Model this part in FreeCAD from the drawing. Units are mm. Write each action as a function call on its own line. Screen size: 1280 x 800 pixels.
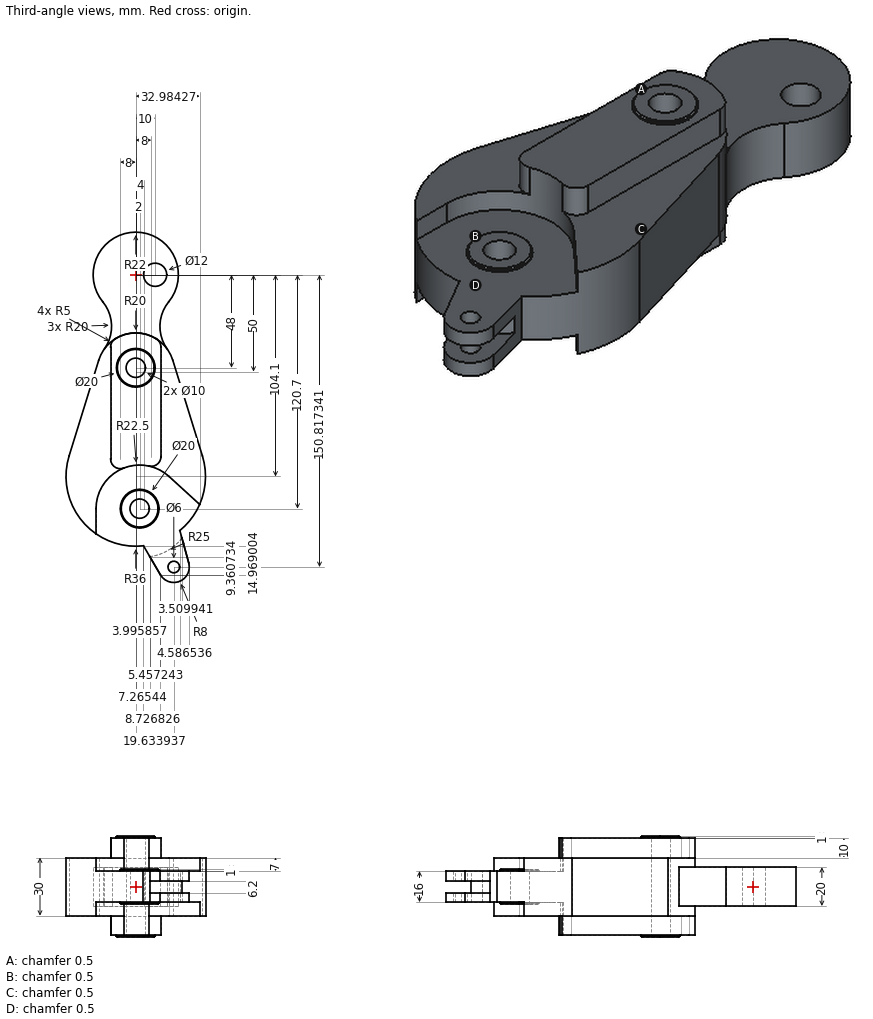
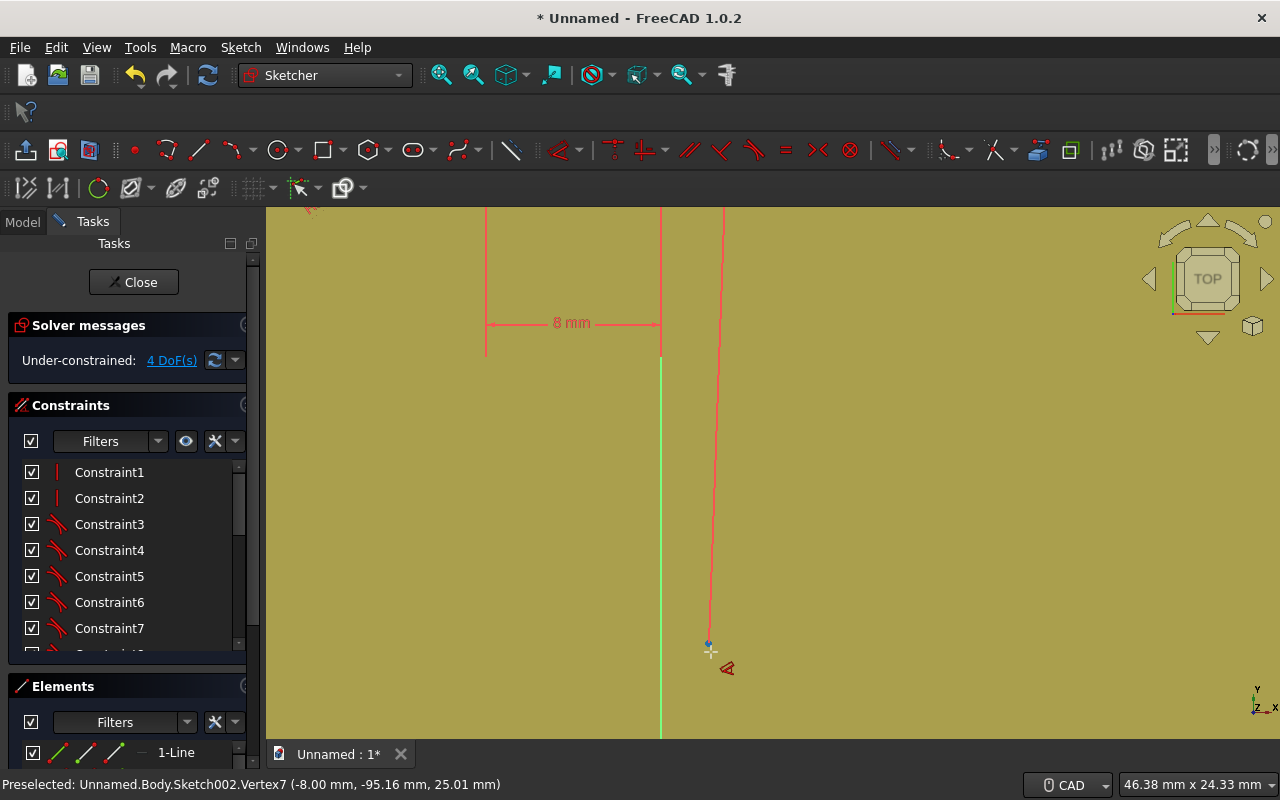
click(709, 643)
click(685, 677)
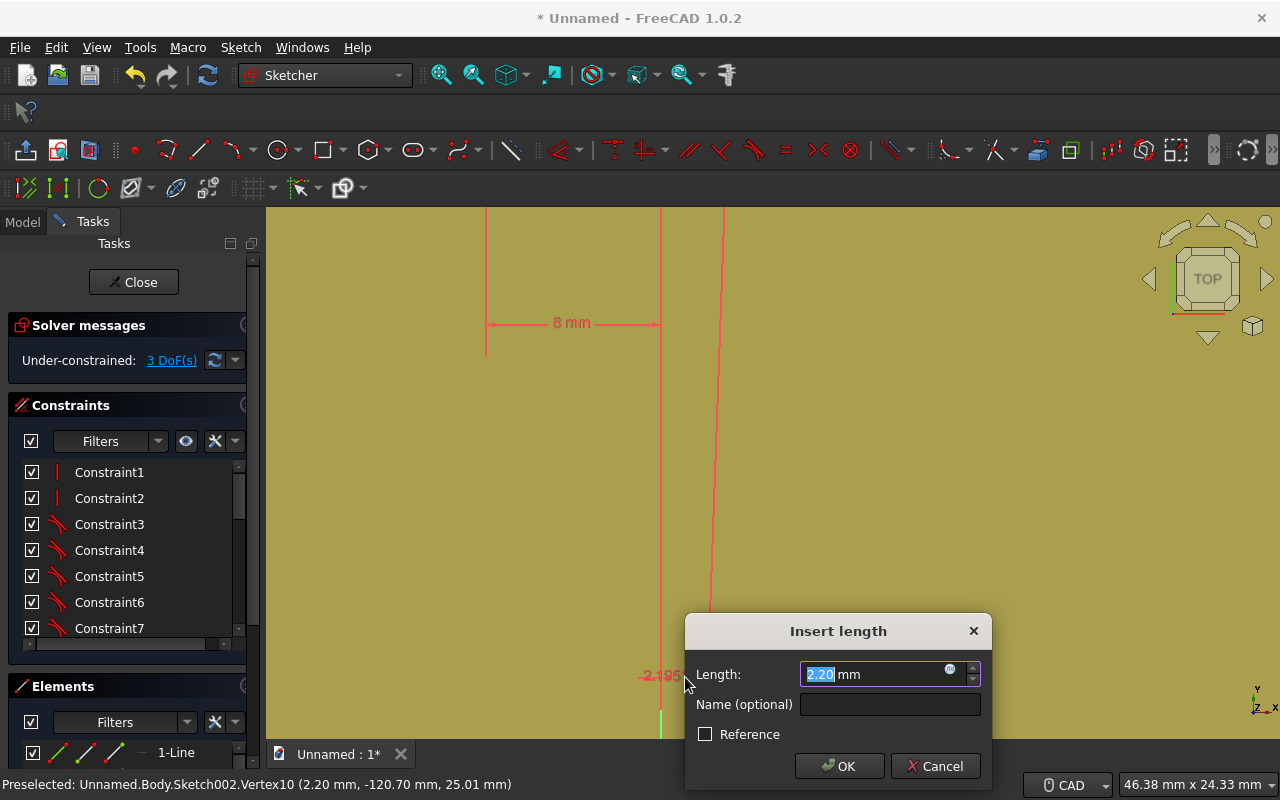
text(2)
key(Return)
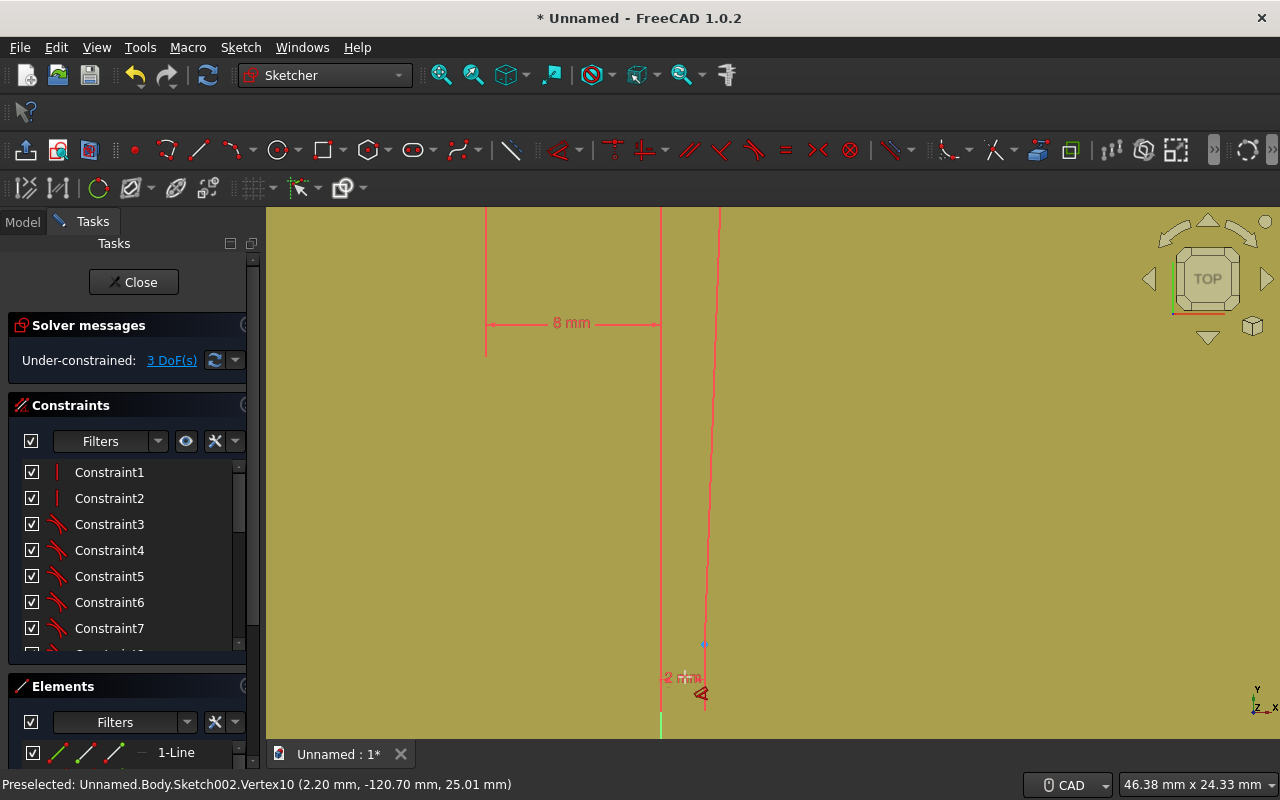
scroll(713, 711, down, 9)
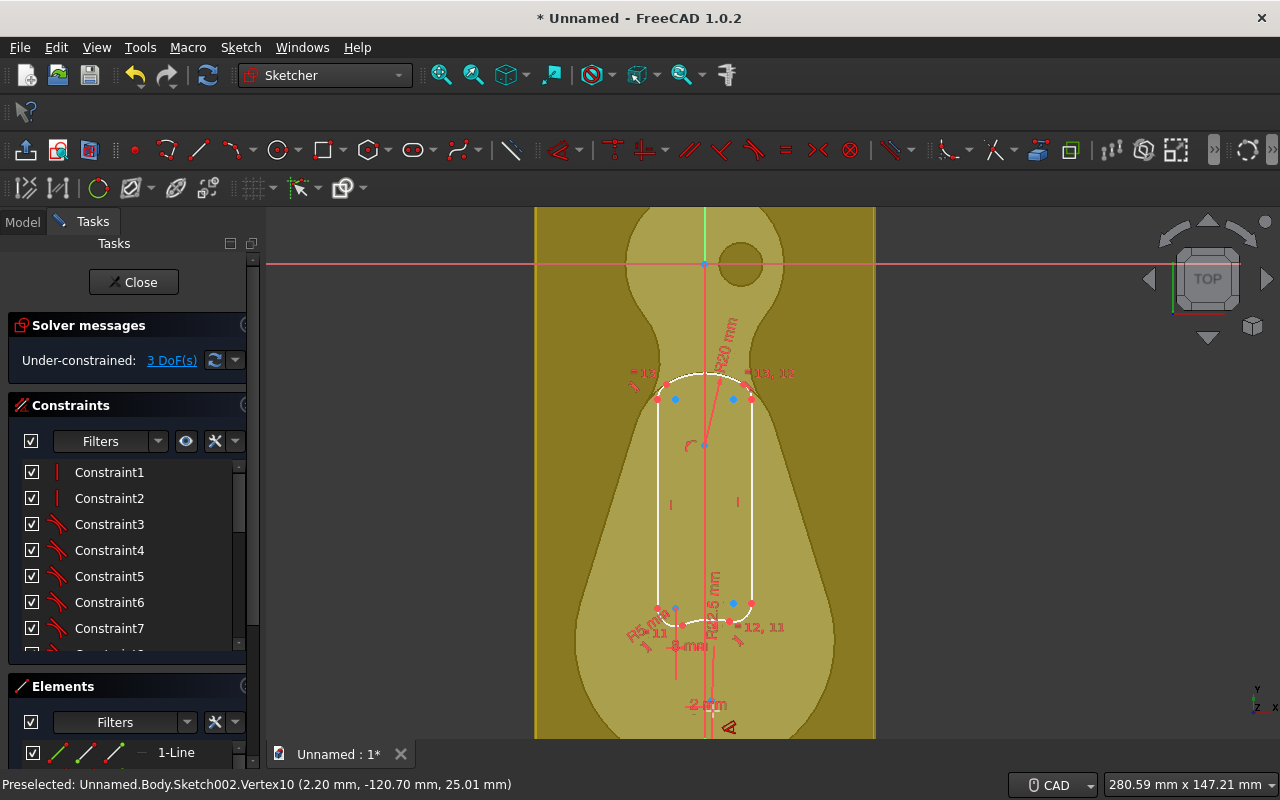
scroll(734, 604, up, 2)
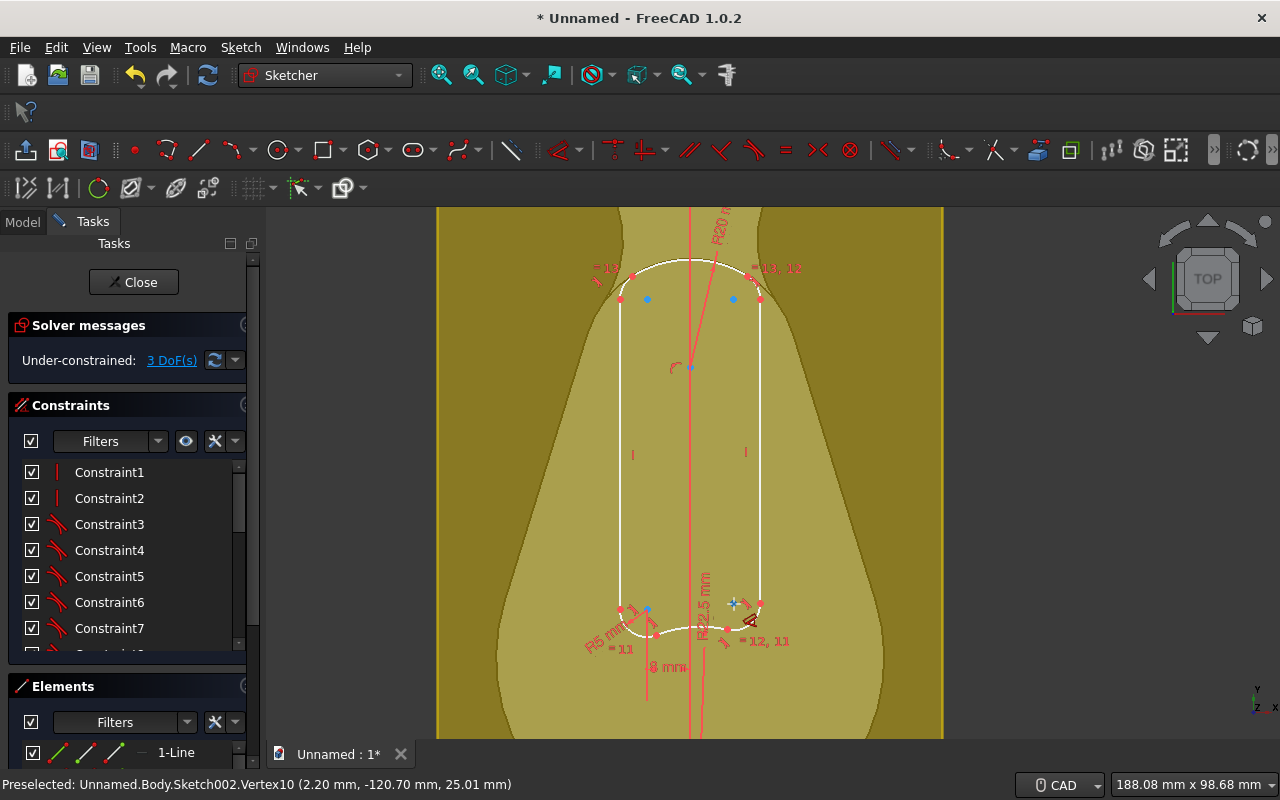
click(733, 603)
click(712, 709)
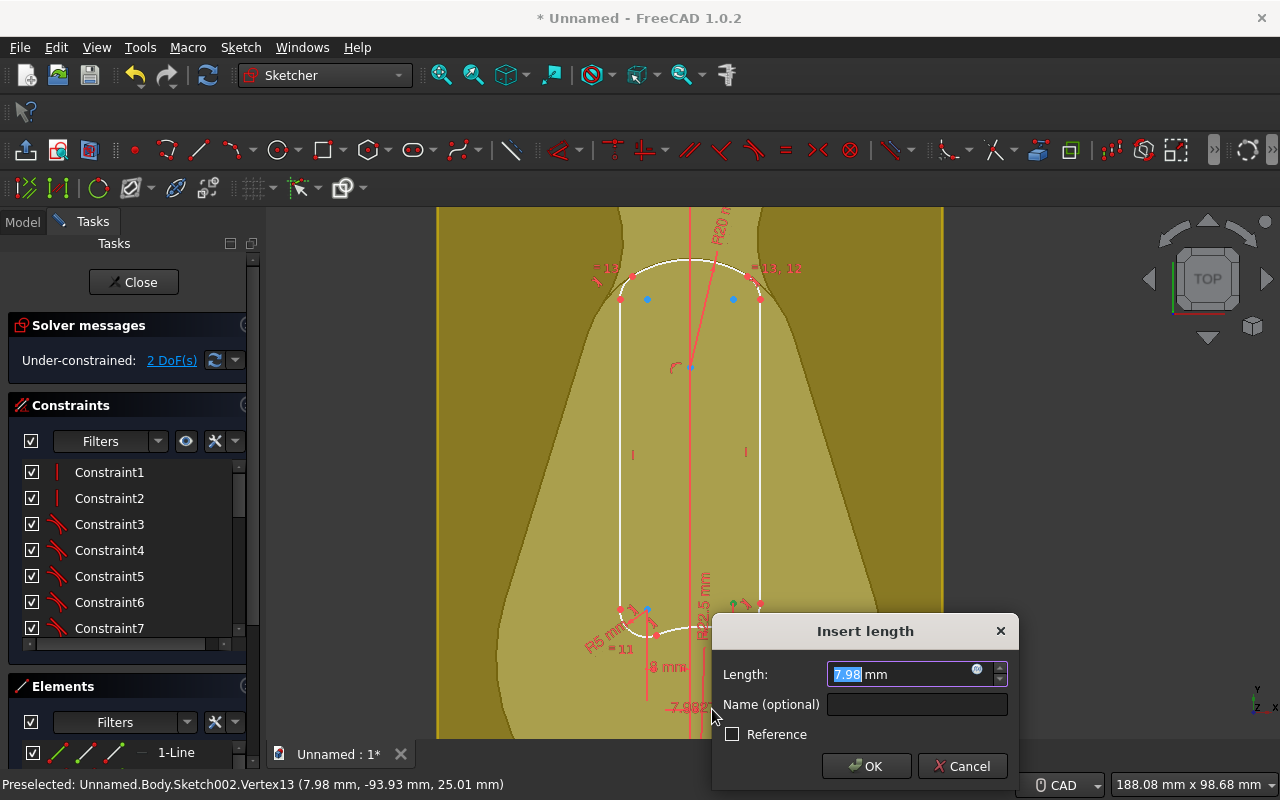
text(8)
key(Return)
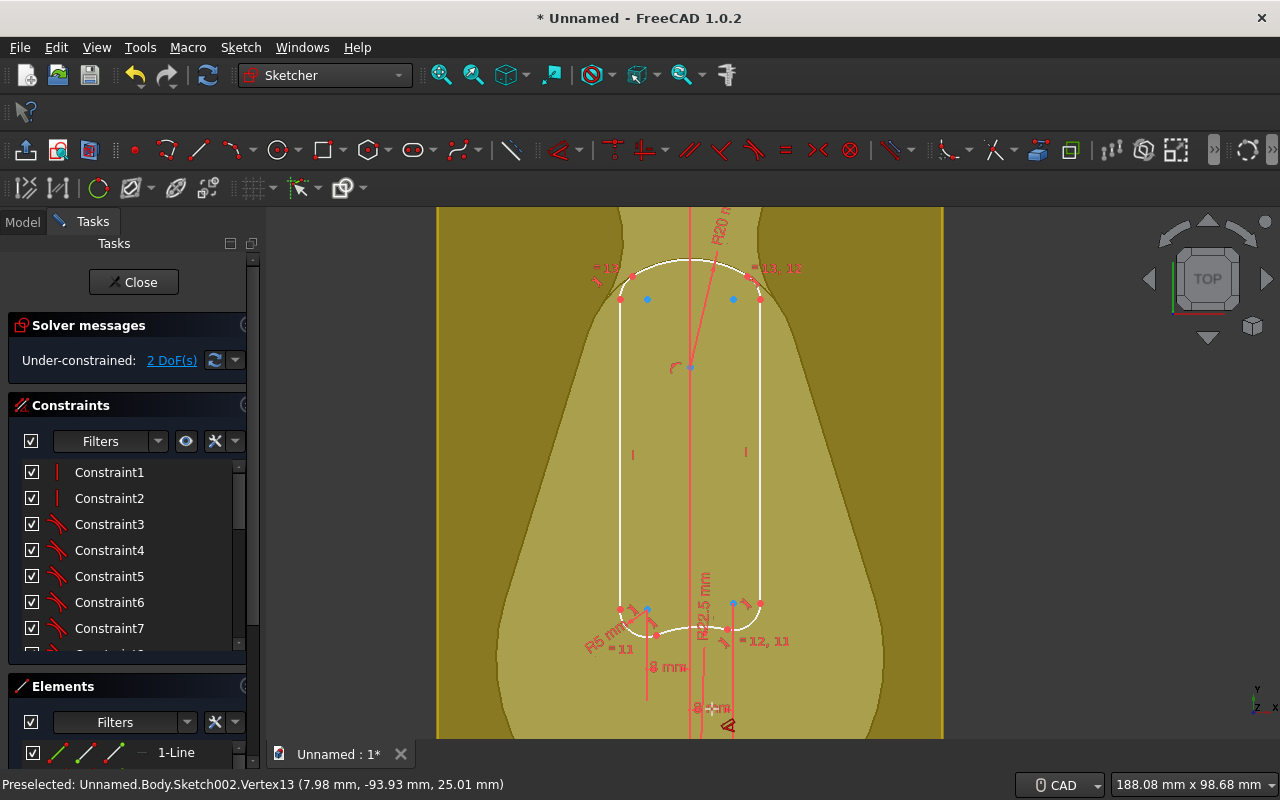
click(690, 368)
click(724, 301)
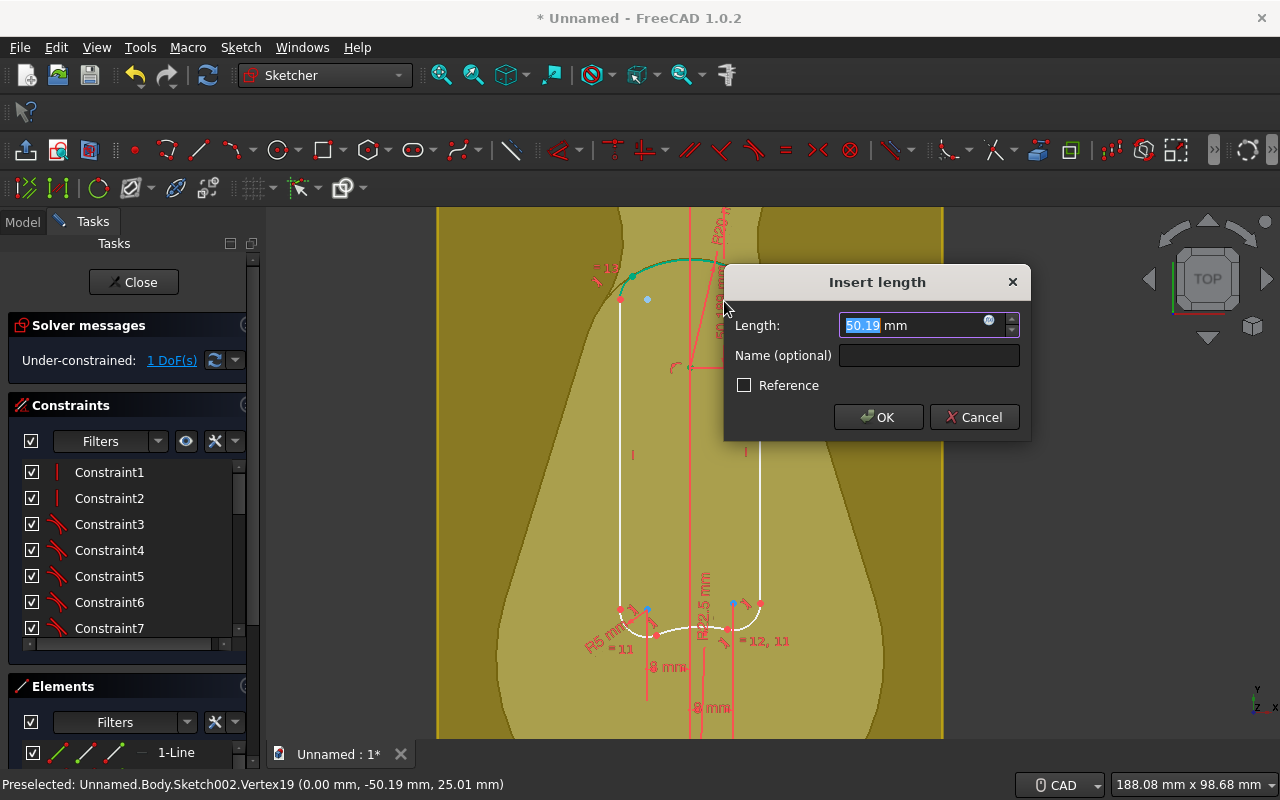
text(50)
key(Return)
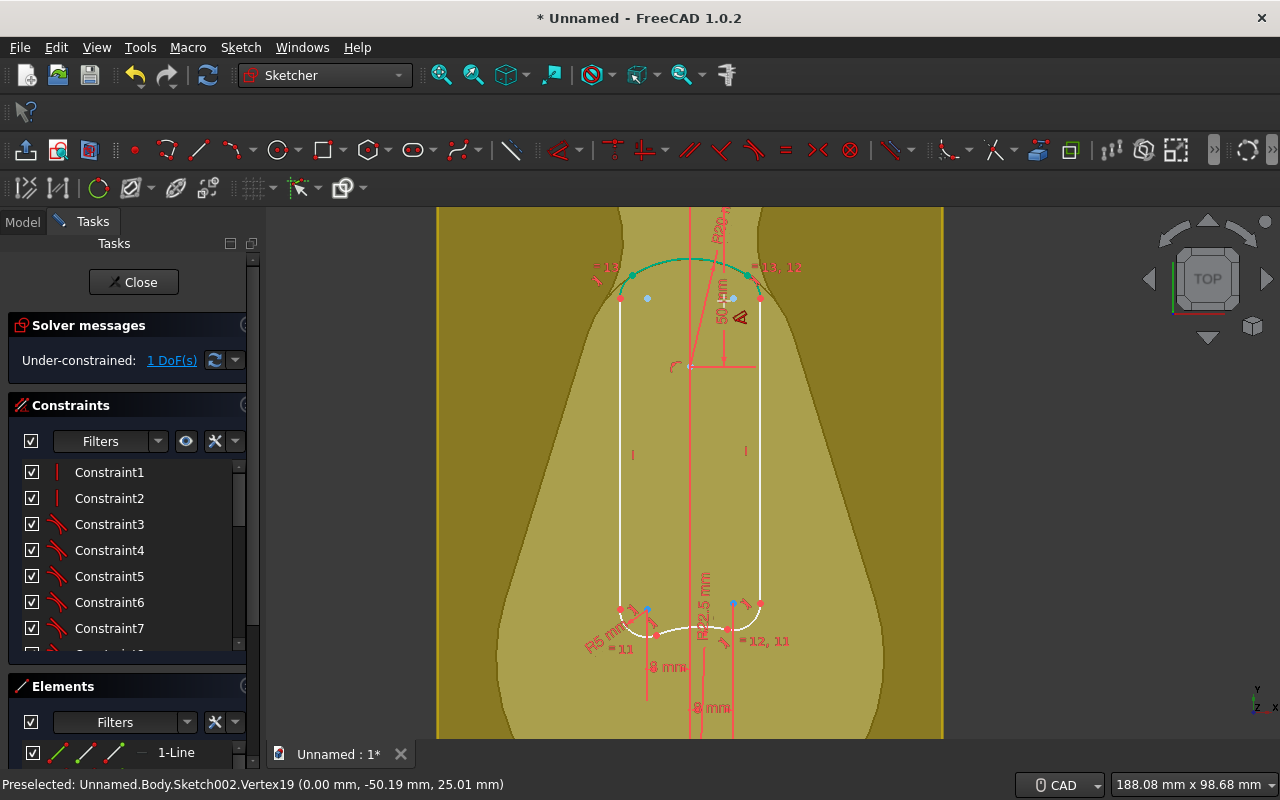
scroll(734, 691, down, 2)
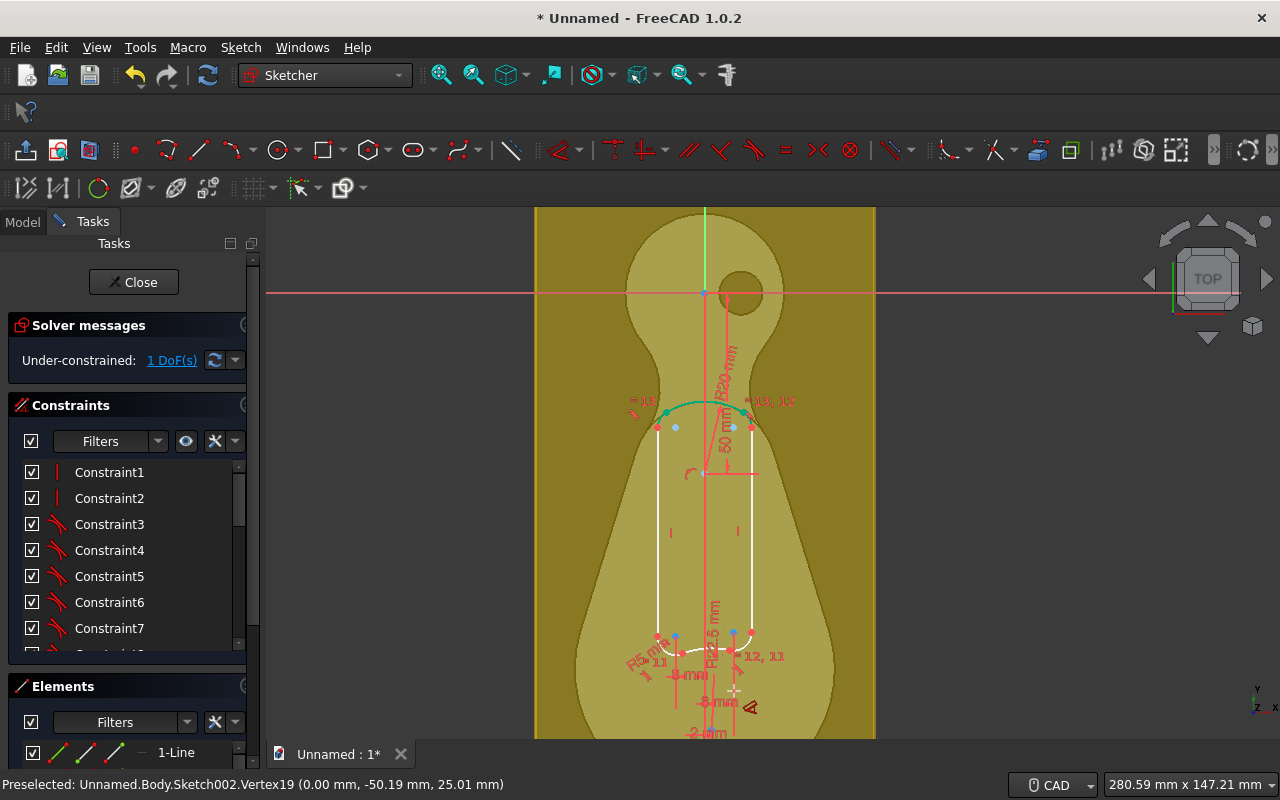
scroll(703, 300, down, 1)